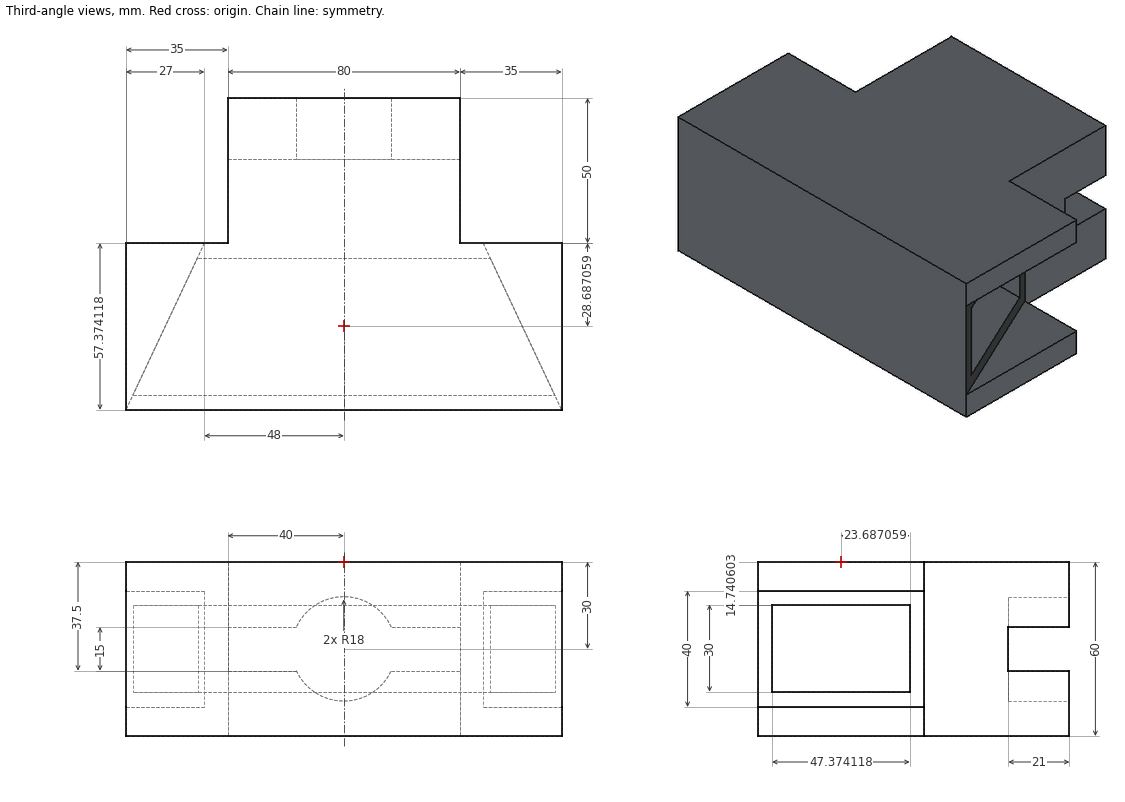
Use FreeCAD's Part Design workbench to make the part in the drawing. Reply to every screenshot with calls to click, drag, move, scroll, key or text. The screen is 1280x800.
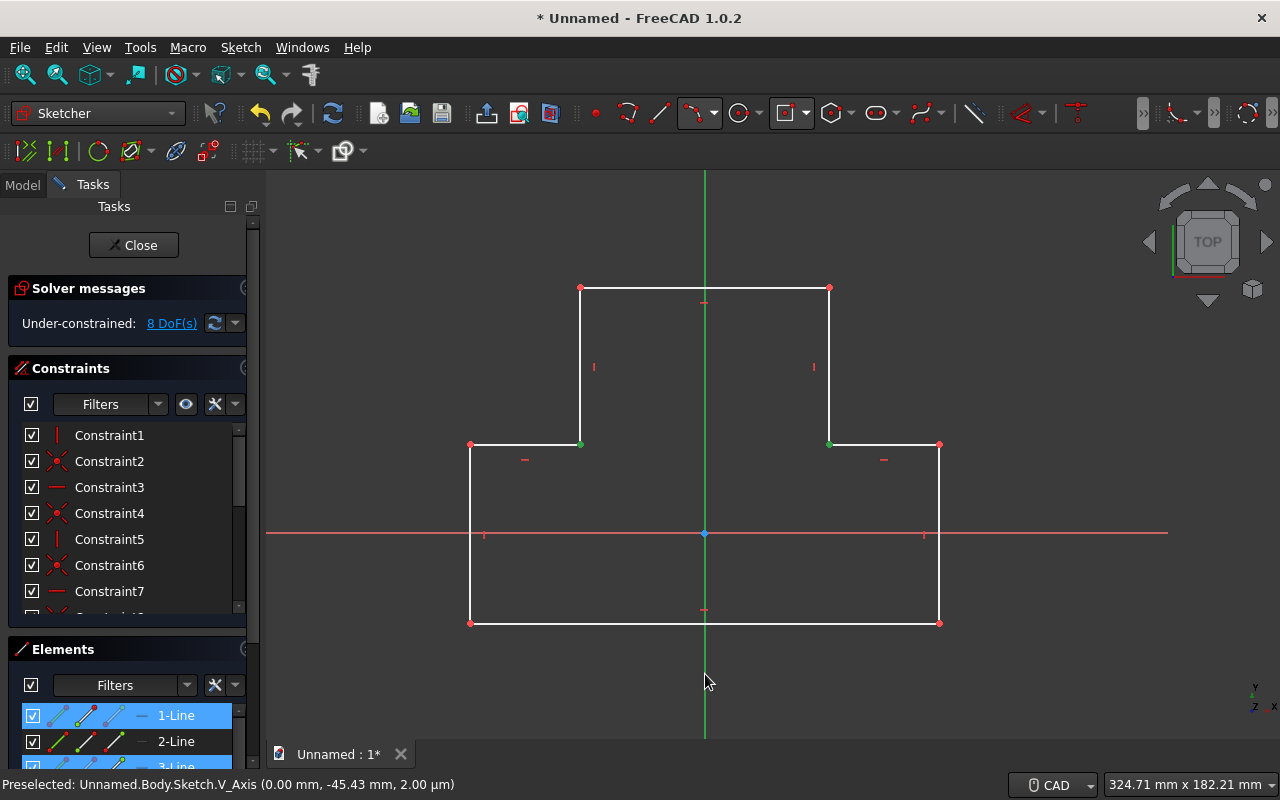
key(s)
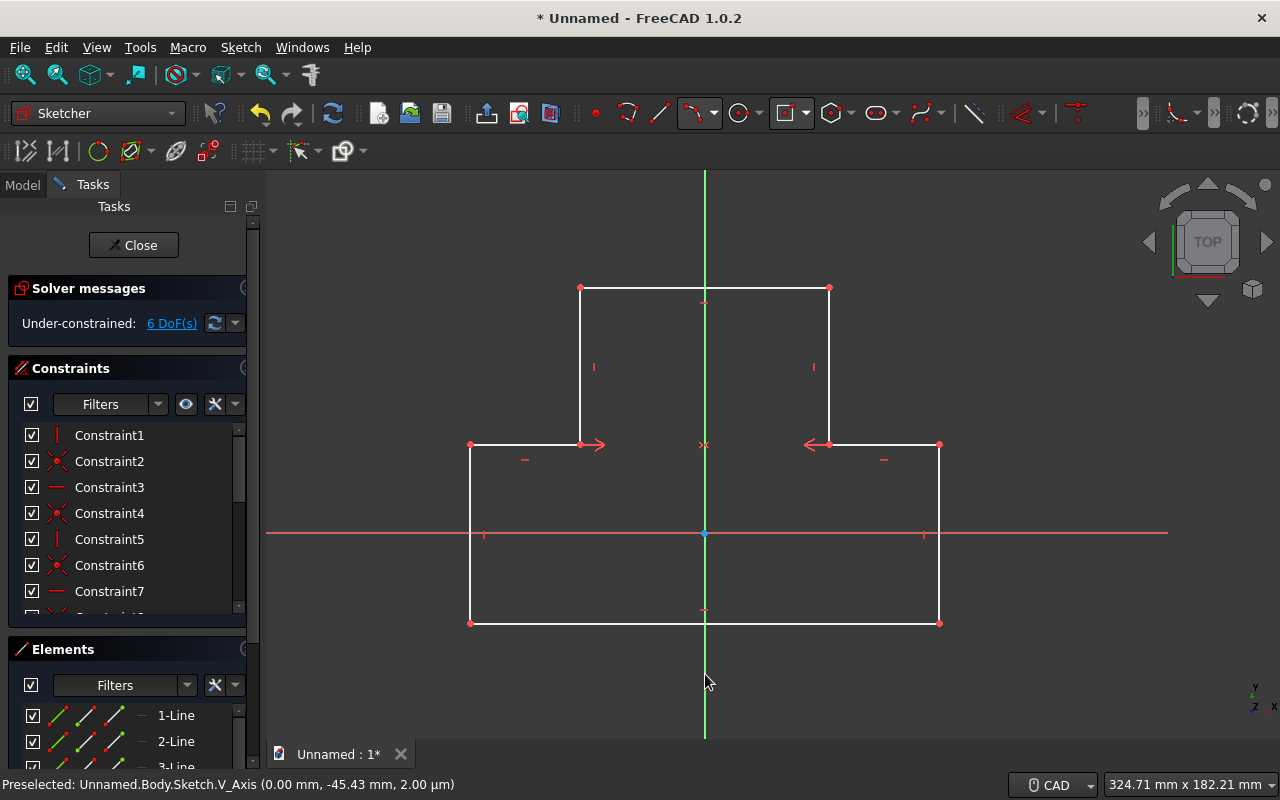
key(d)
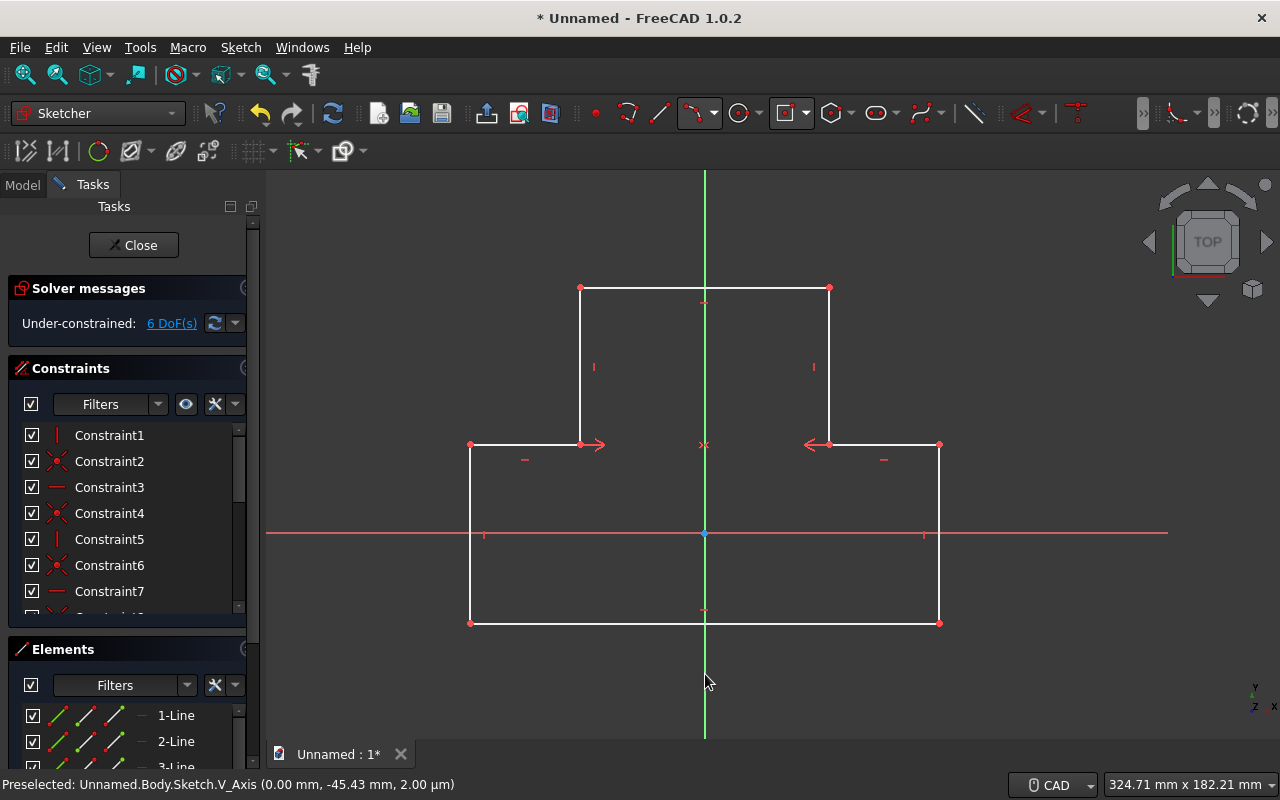
click(829, 398)
click(863, 366)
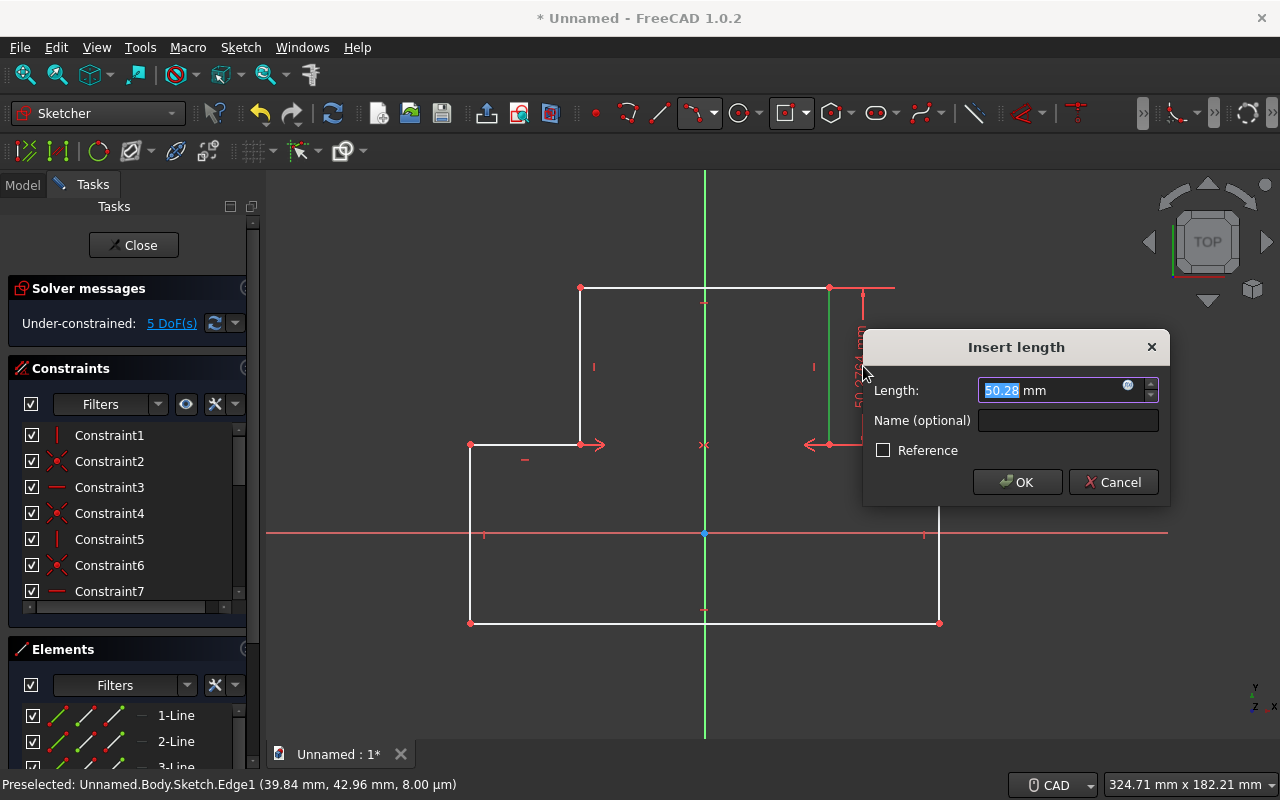
text(50)
key(Return)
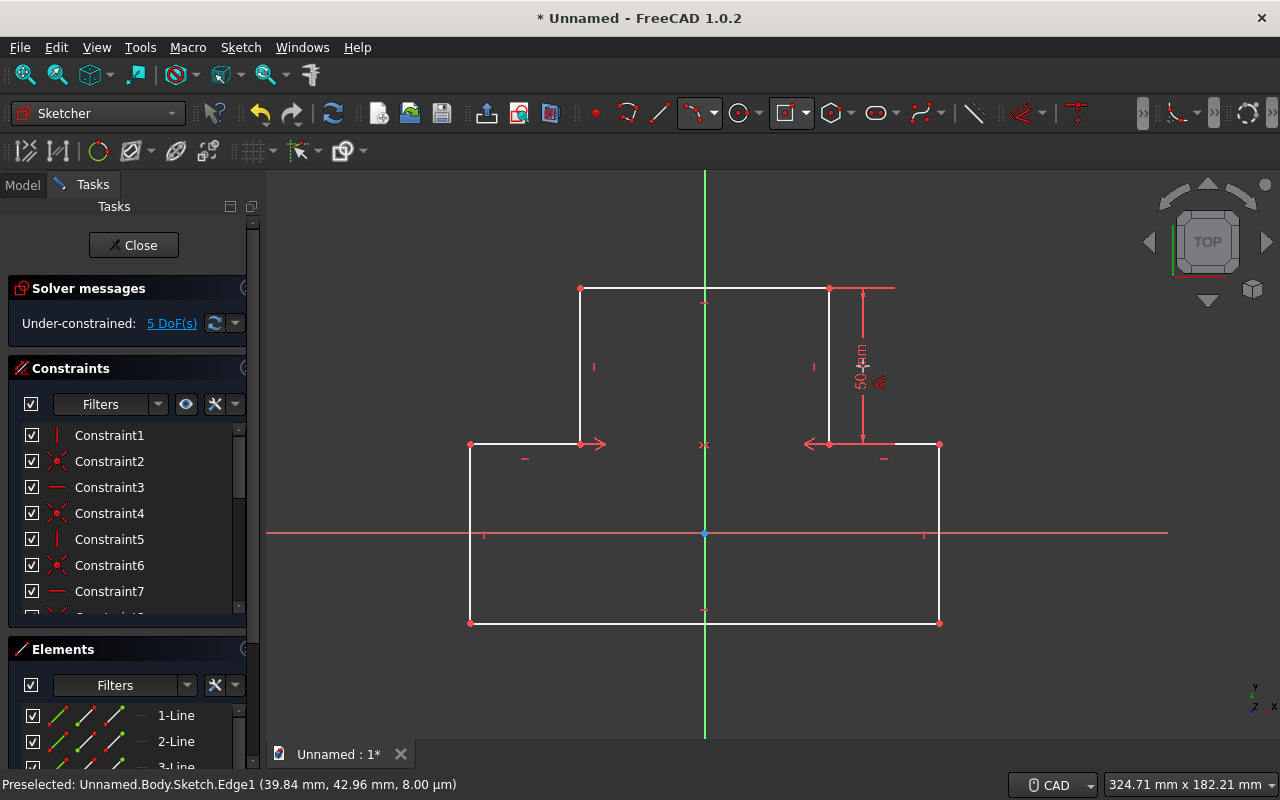
click(754, 288)
click(647, 254)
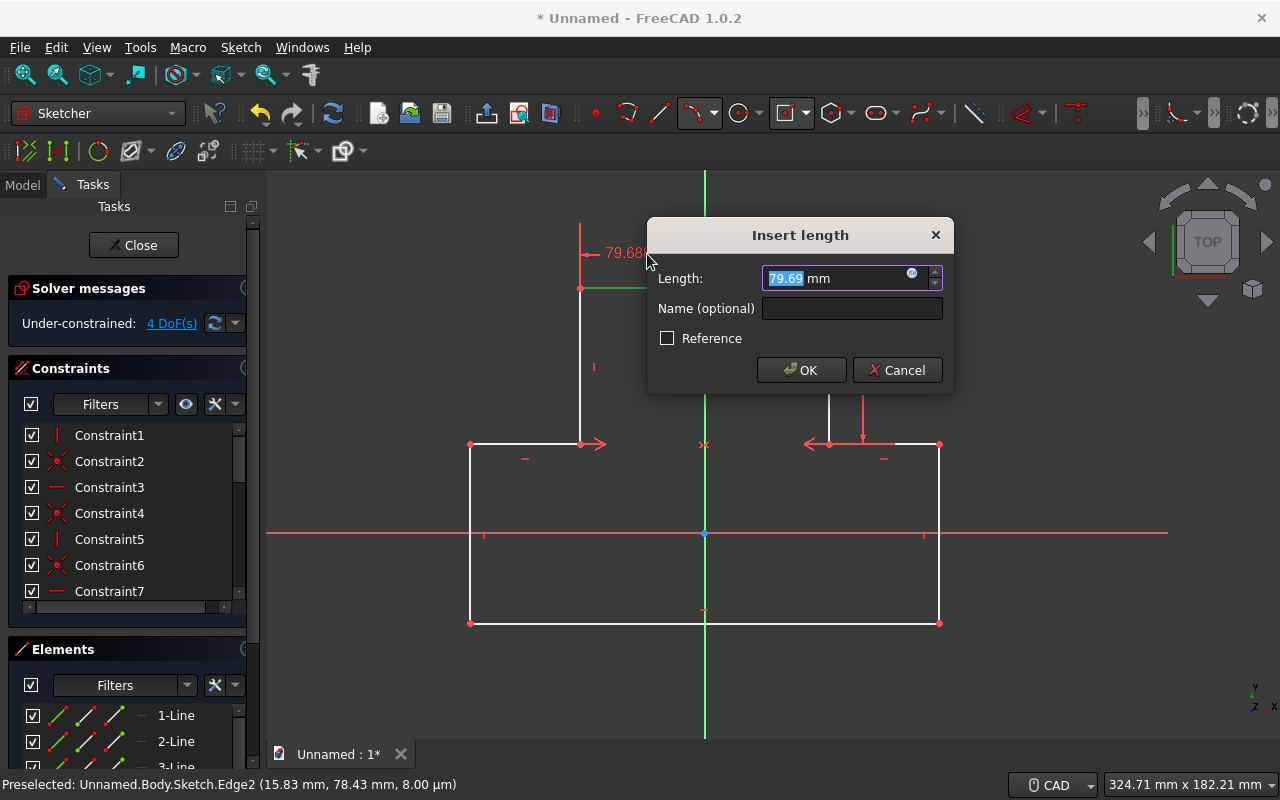
text(80)
key(Return)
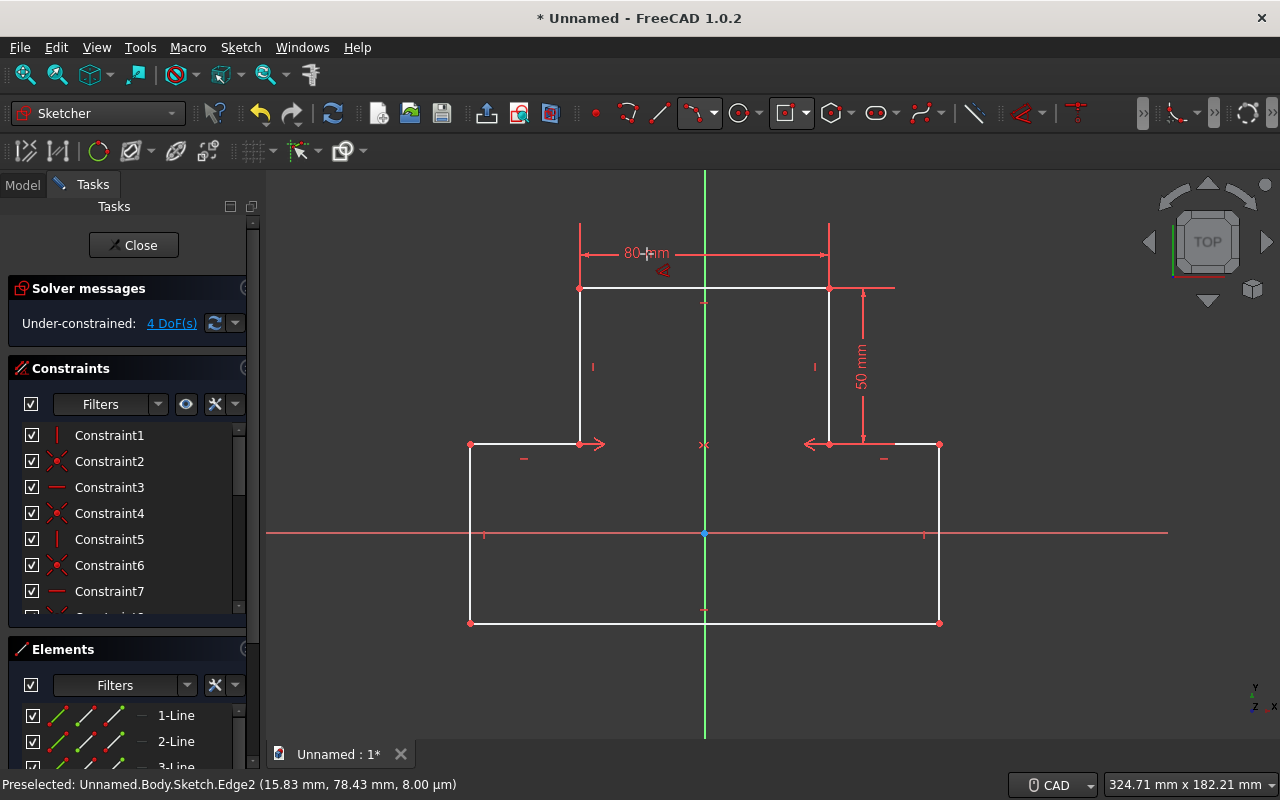
click(547, 444)
click(525, 410)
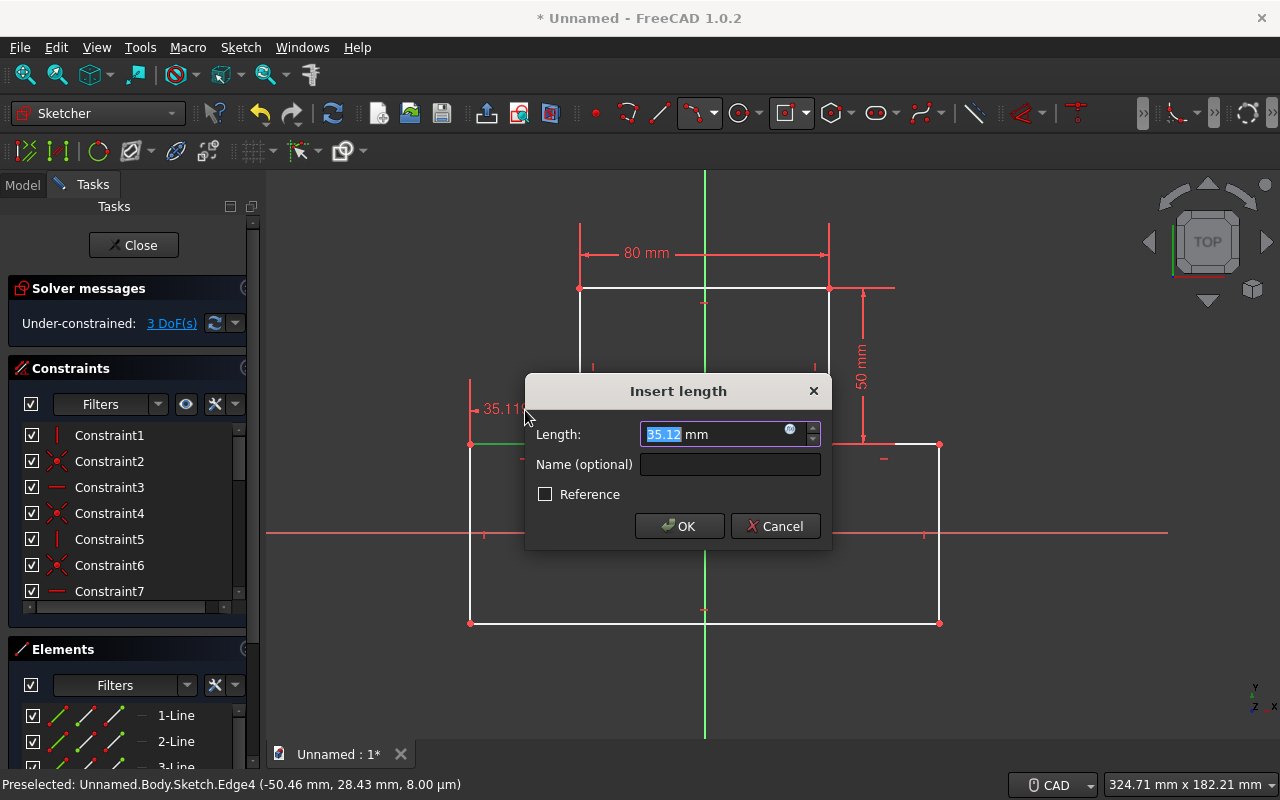
text(35)
key(Return)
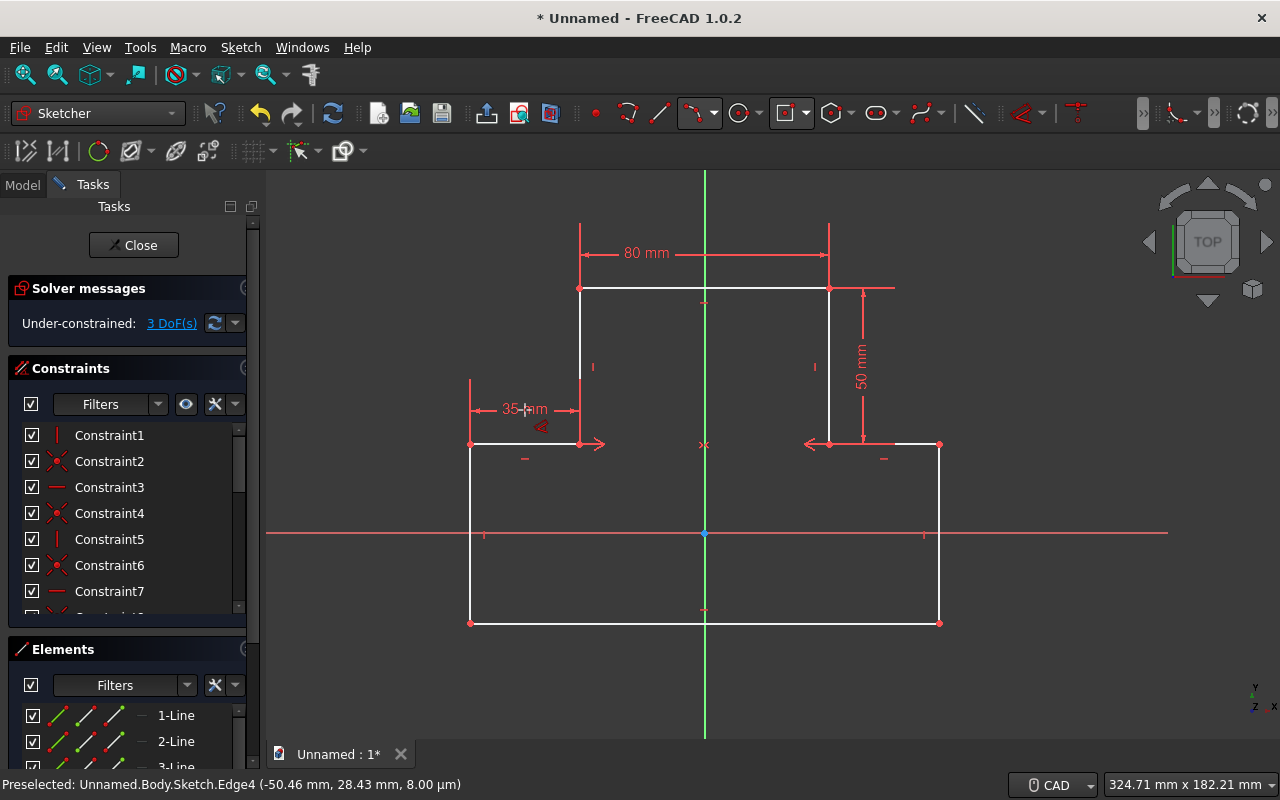
click(906, 444)
click(884, 410)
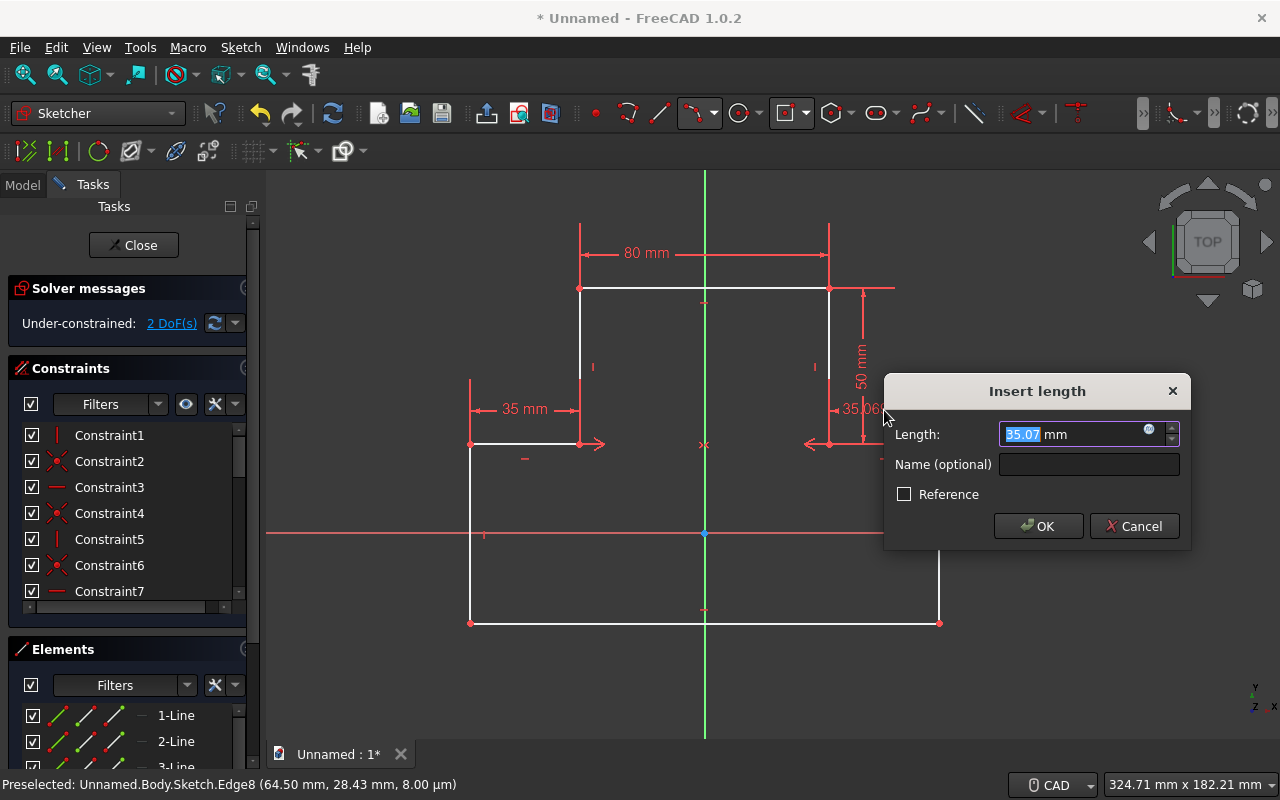
text(35)
key(Return)